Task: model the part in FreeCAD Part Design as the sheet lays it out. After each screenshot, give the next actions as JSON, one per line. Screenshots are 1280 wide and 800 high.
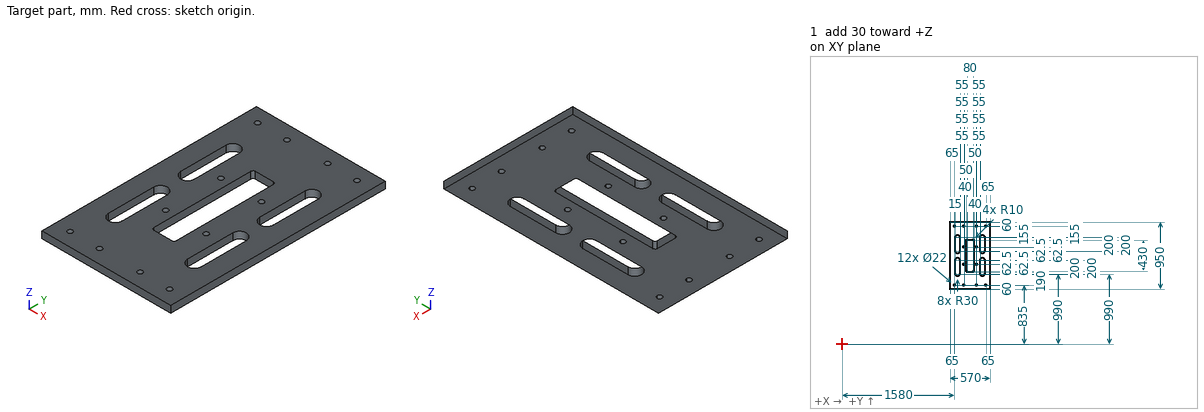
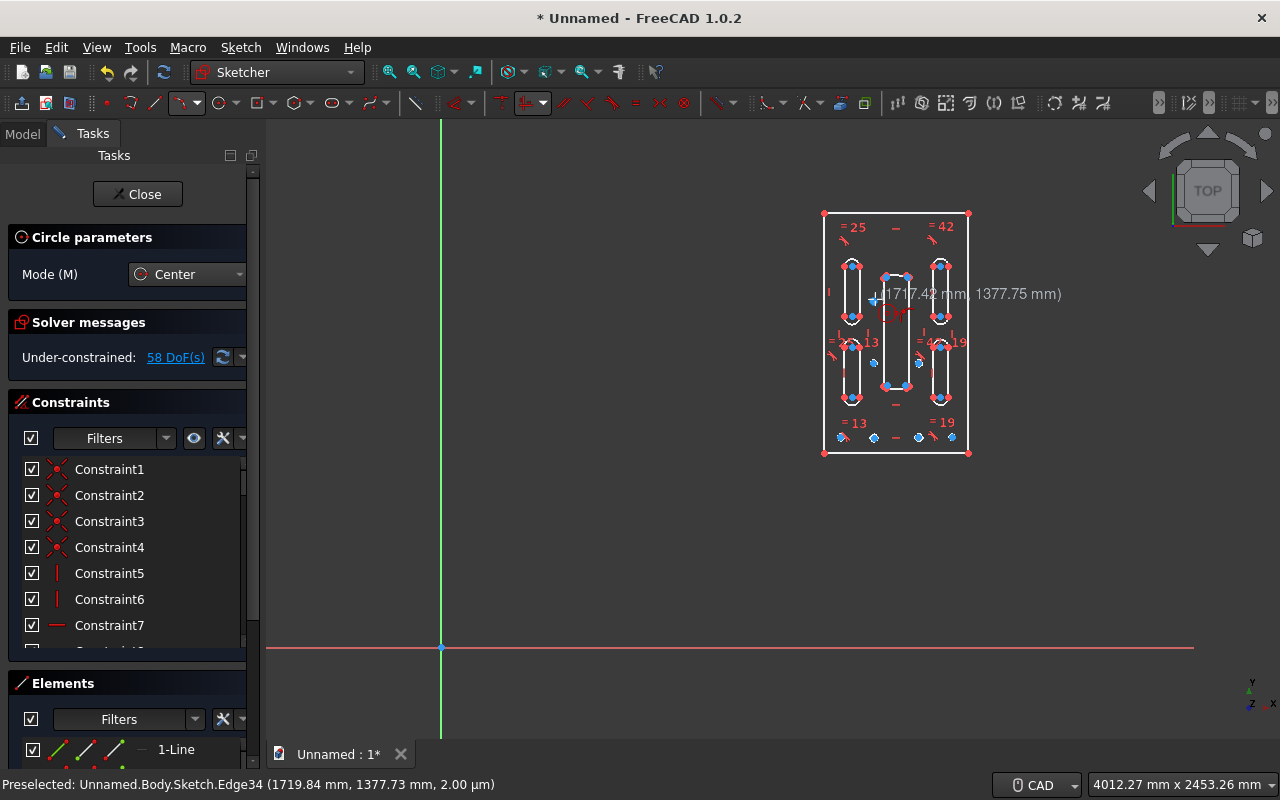
{"action": "scroll", "coordinate": [841, 227], "scroll_direction": "up", "scroll_amount": 11}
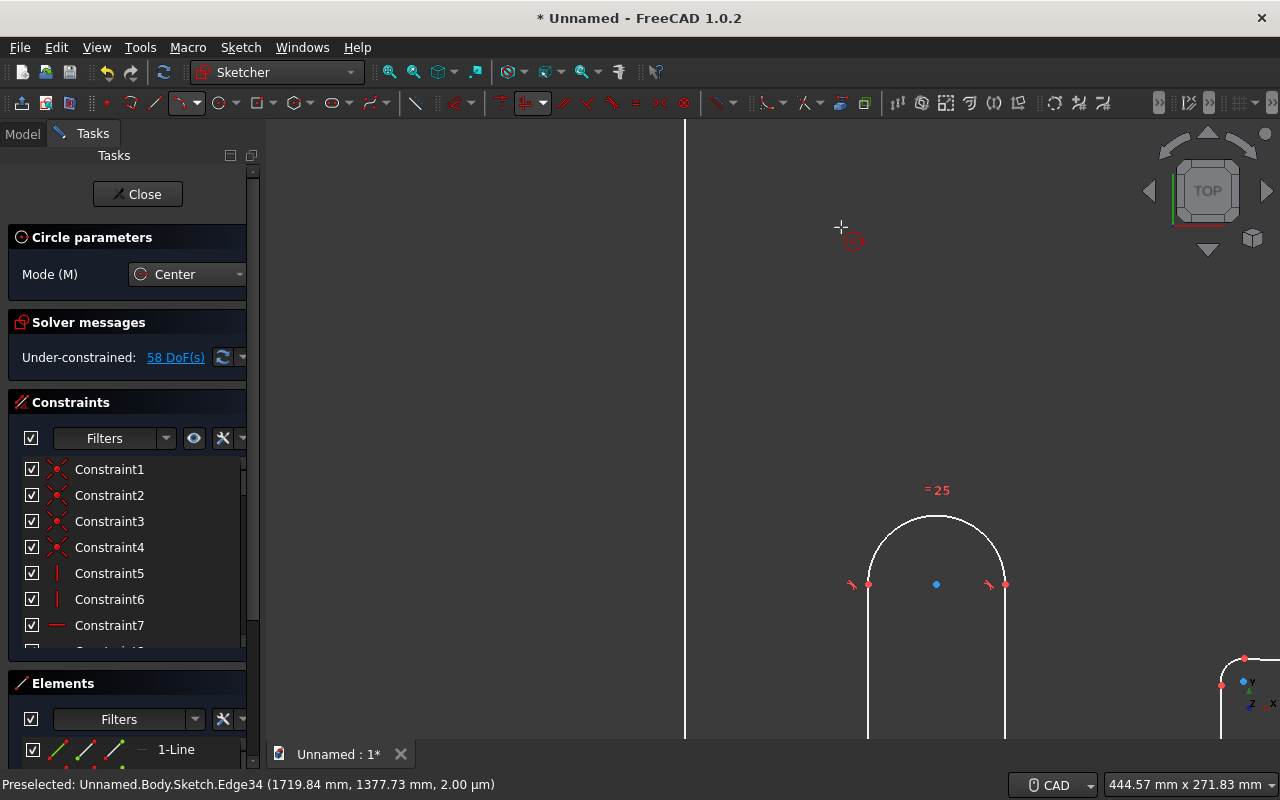
{"action": "scroll", "coordinate": [841, 226], "scroll_direction": "down", "scroll_amount": 11}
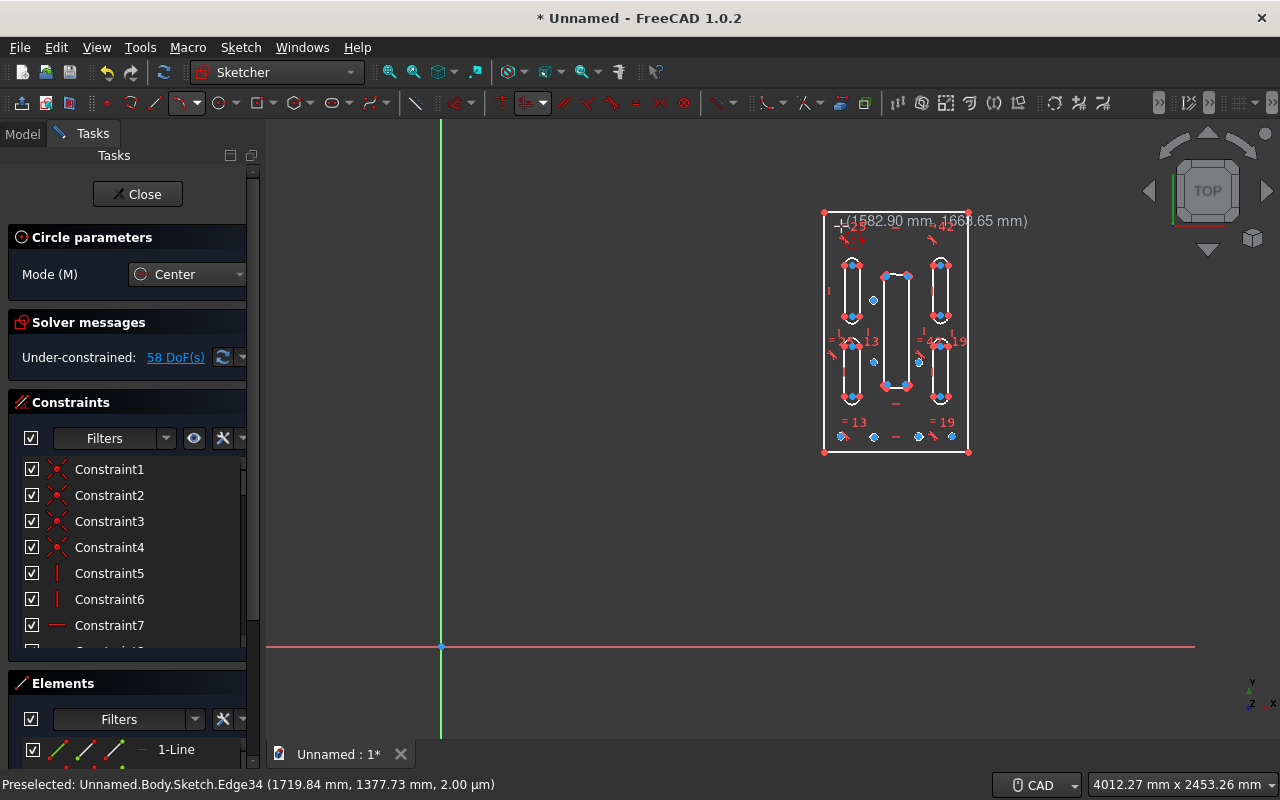
{"action": "left_click", "coordinate": [841, 226]}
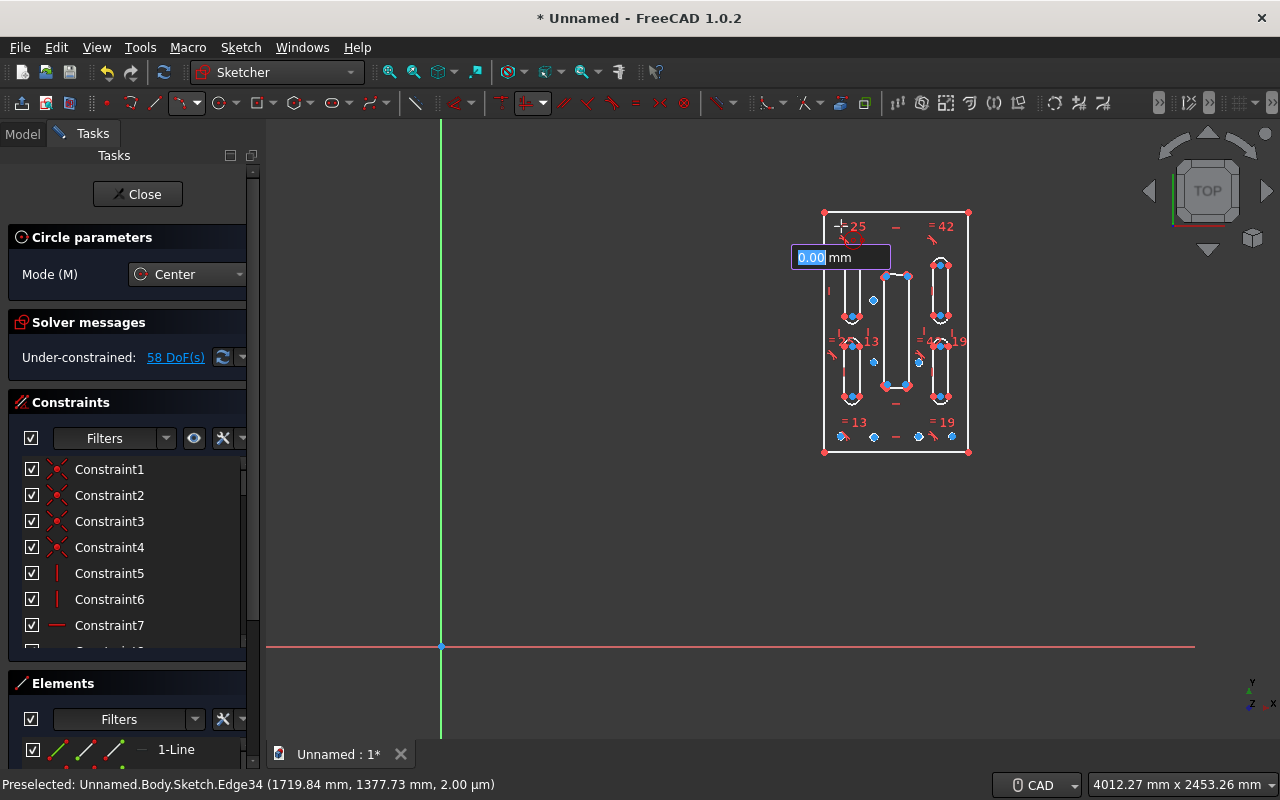
{"action": "scroll", "coordinate": [843, 228], "scroll_direction": "up", "scroll_amount": 9}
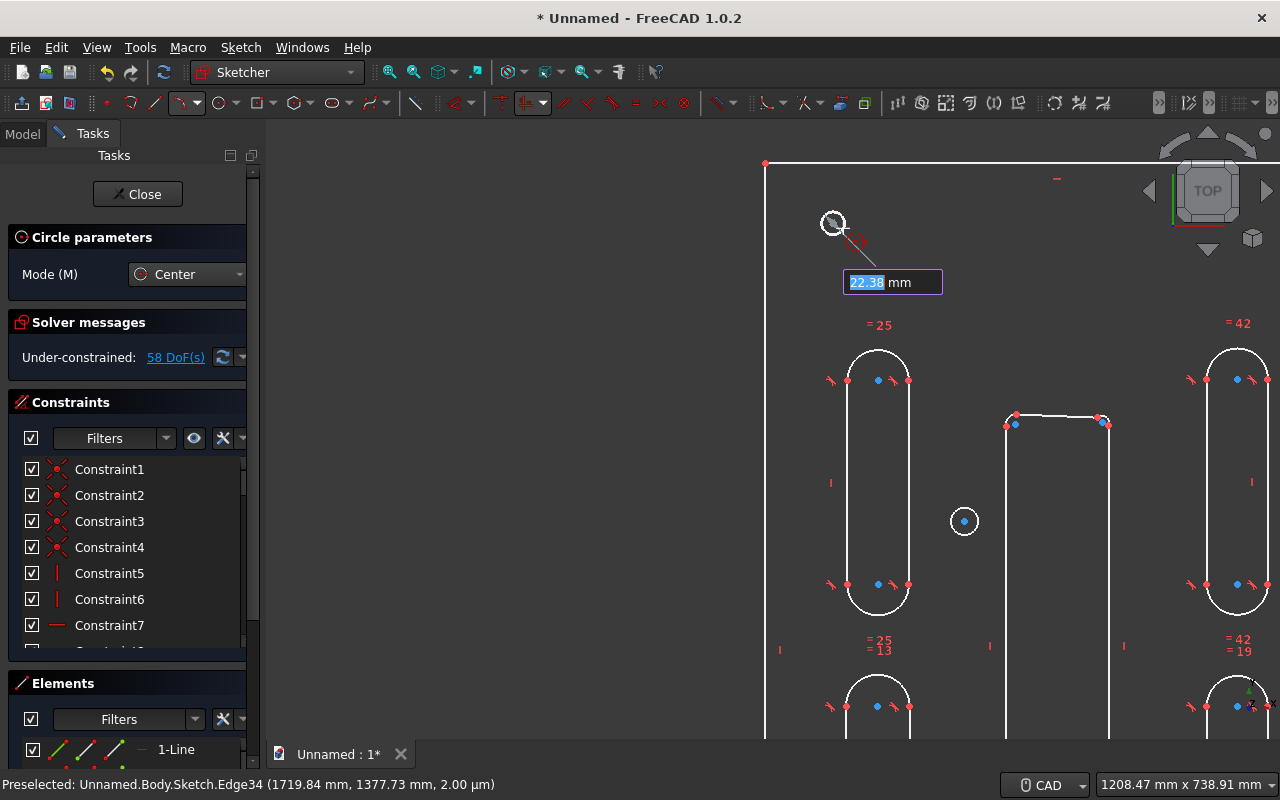
{"action": "left_click", "coordinate": [839, 226]}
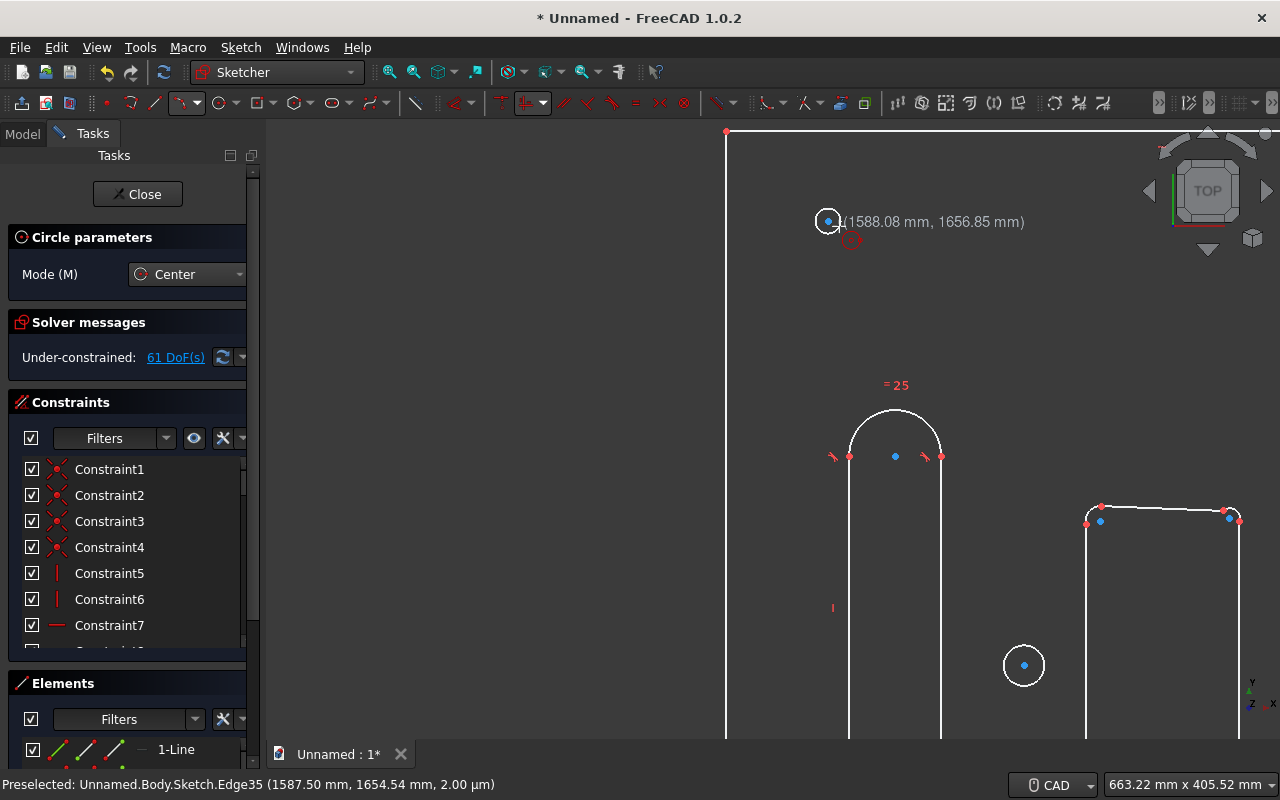
{"action": "scroll", "coordinate": [1025, 215], "scroll_direction": "up", "scroll_amount": 2}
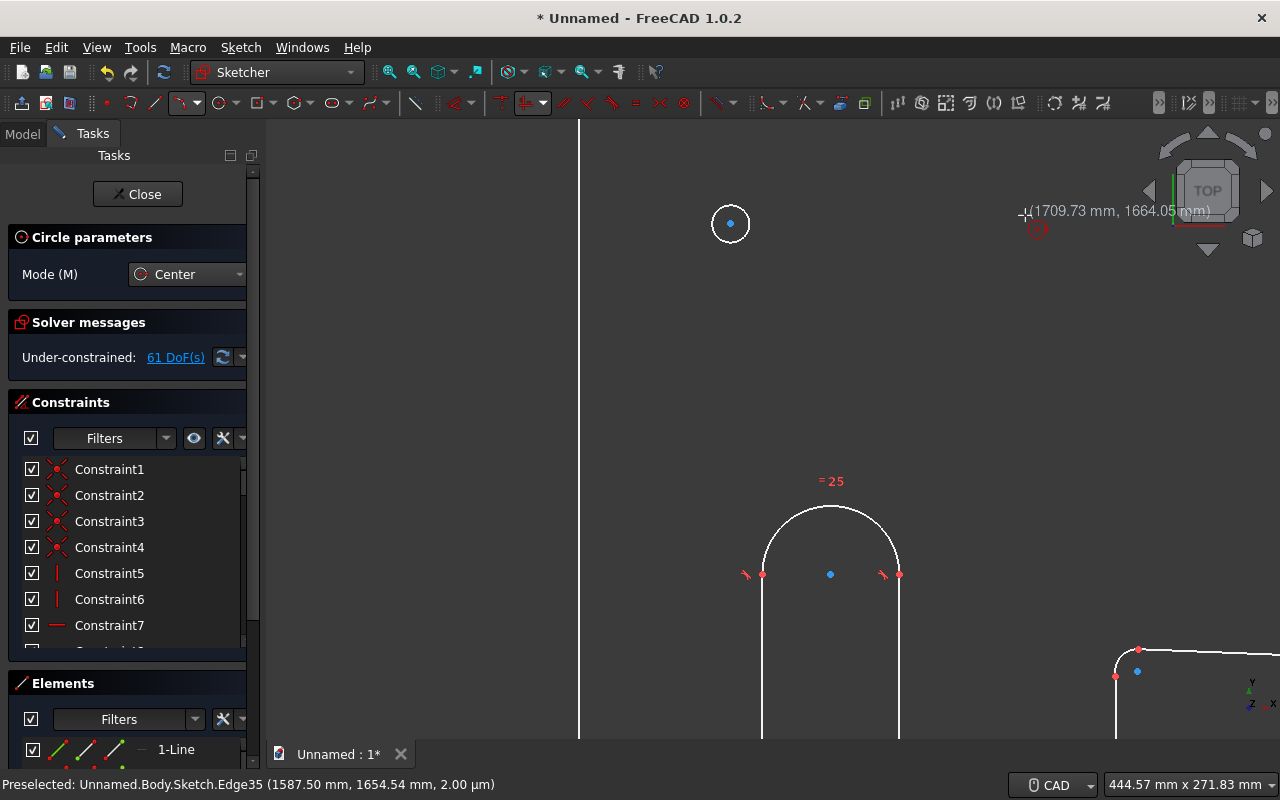
{"action": "scroll", "coordinate": [854, 228], "scroll_direction": "down", "scroll_amount": 11}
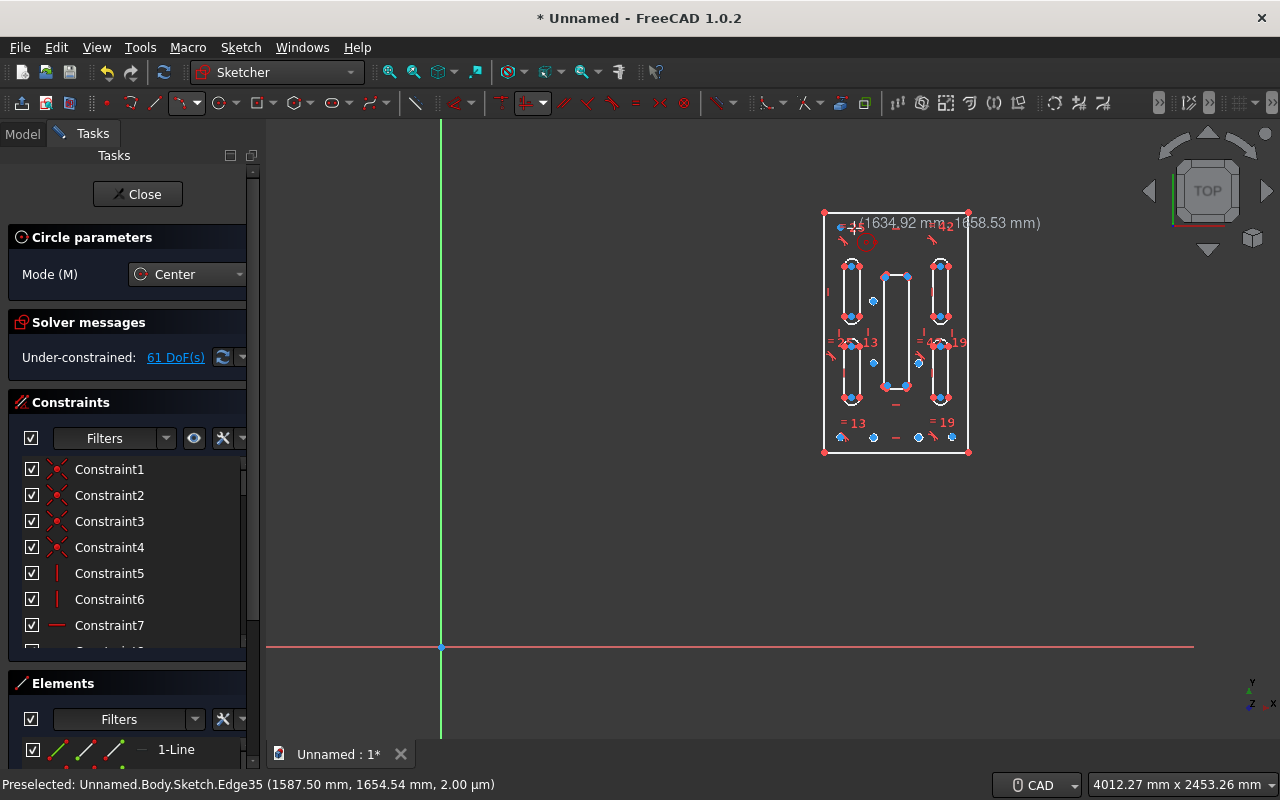
{"action": "left_click", "coordinate": [873, 227]}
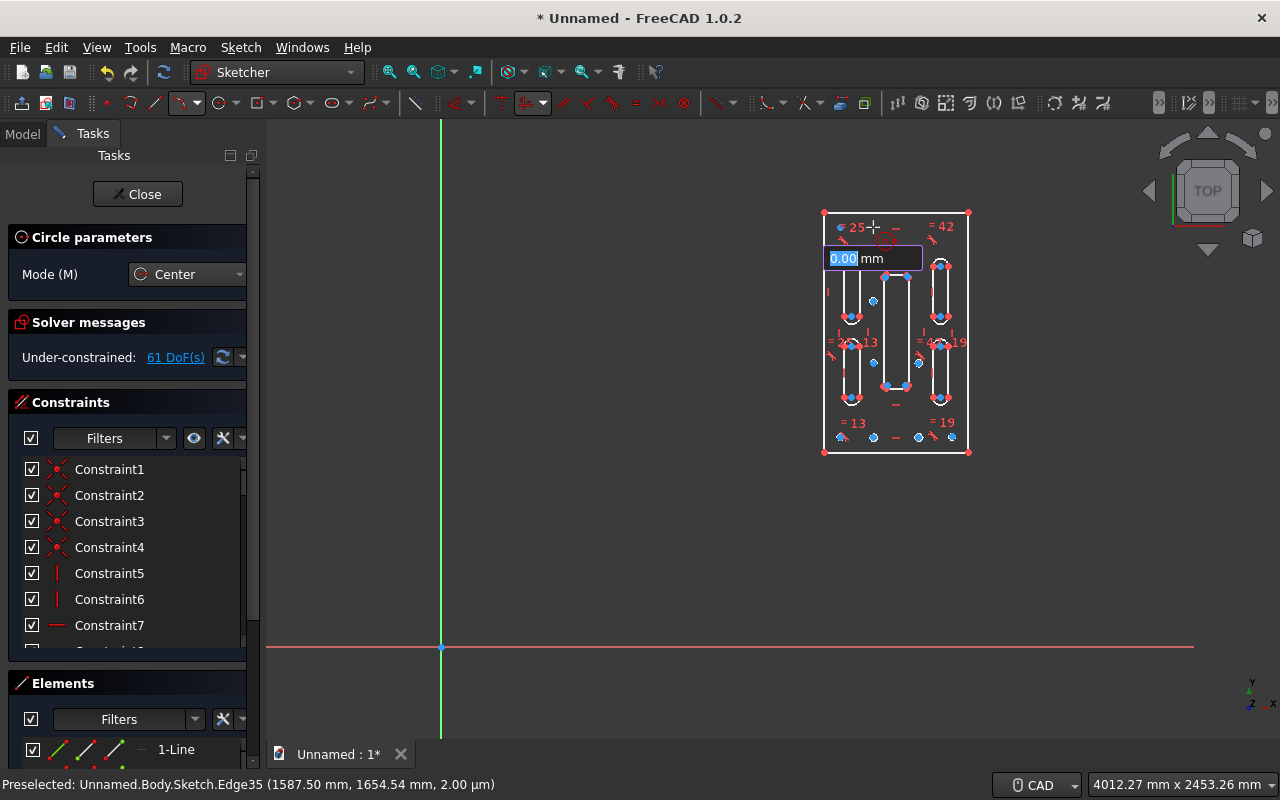
{"action": "scroll", "coordinate": [875, 229], "scroll_direction": "up", "scroll_amount": 9}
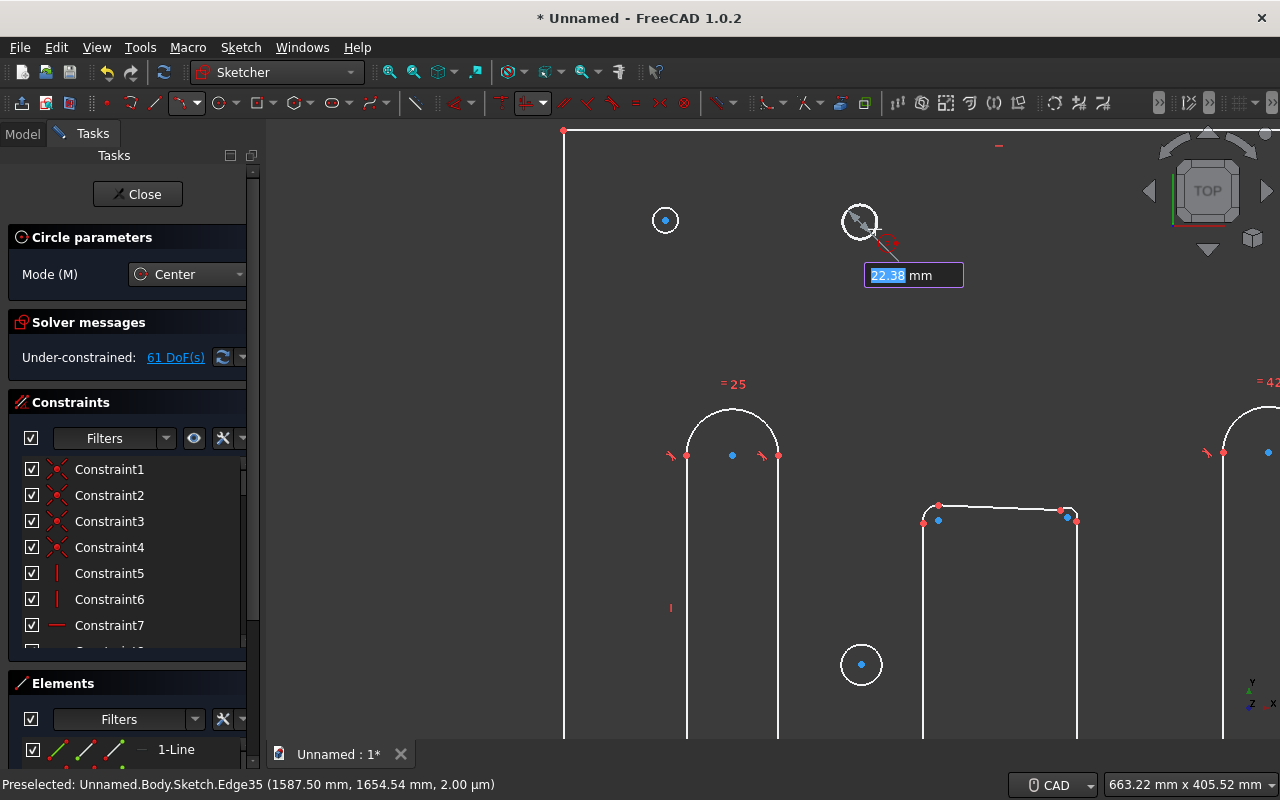
{"action": "left_click", "coordinate": [875, 226]}